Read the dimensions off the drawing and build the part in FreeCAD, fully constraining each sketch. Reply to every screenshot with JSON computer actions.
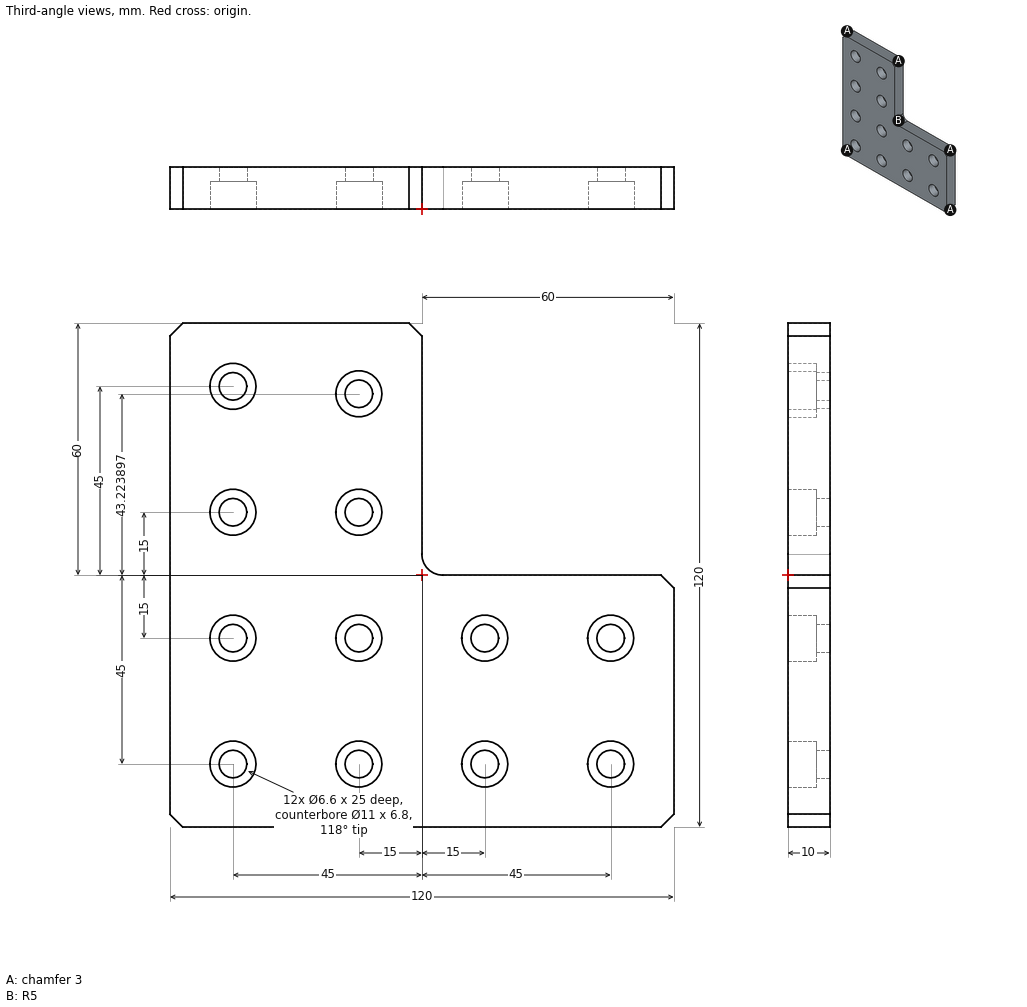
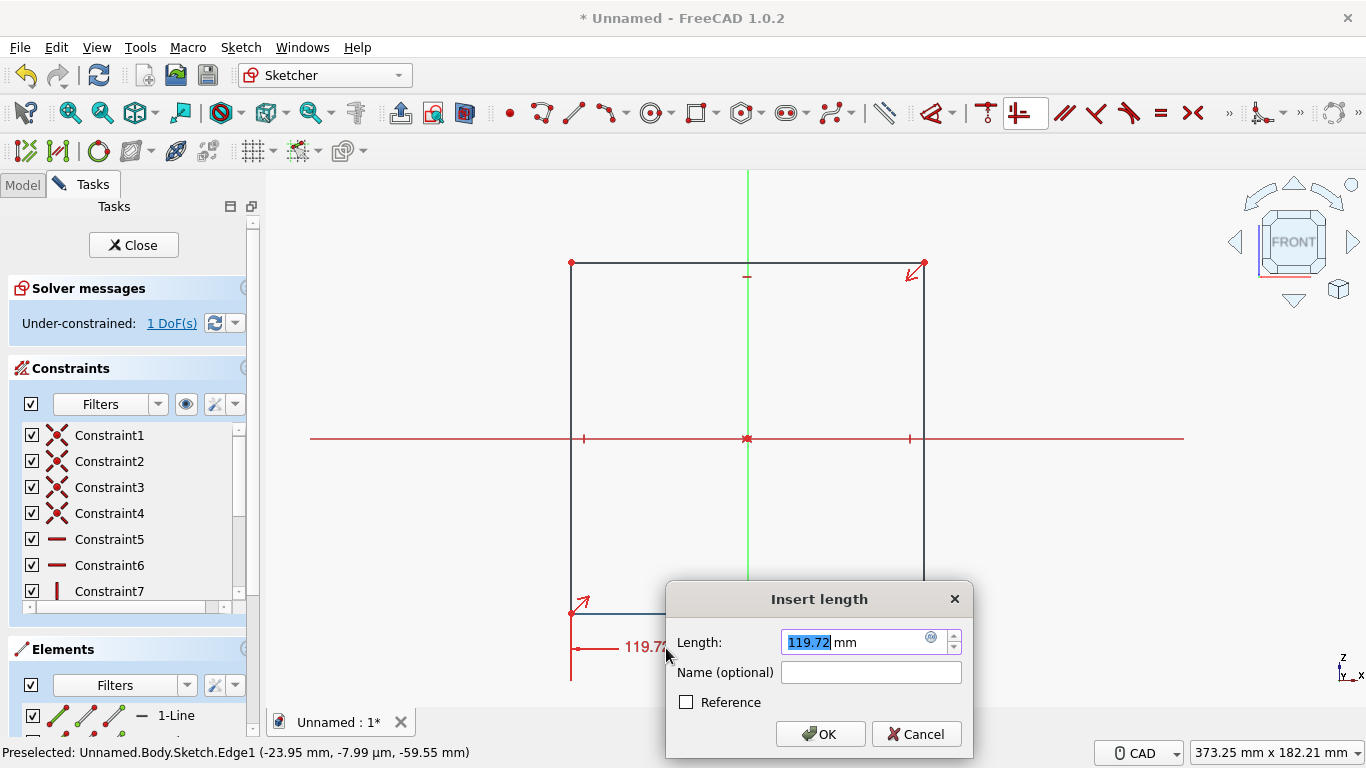
{"action": "type", "text": "120"}
{"action": "key", "text": "Return"}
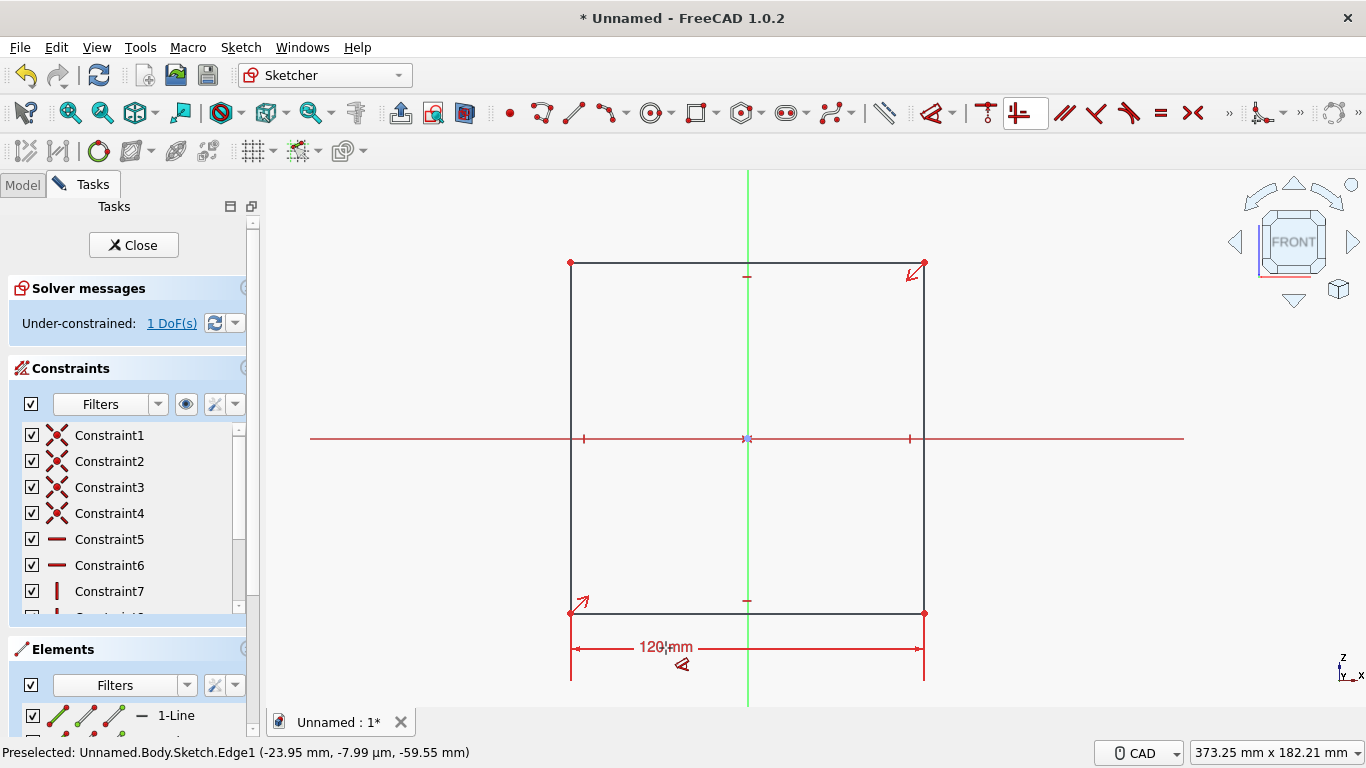
{"action": "left_click", "coordinate": [924, 509]}
{"action": "left_click", "coordinate": [958, 358]}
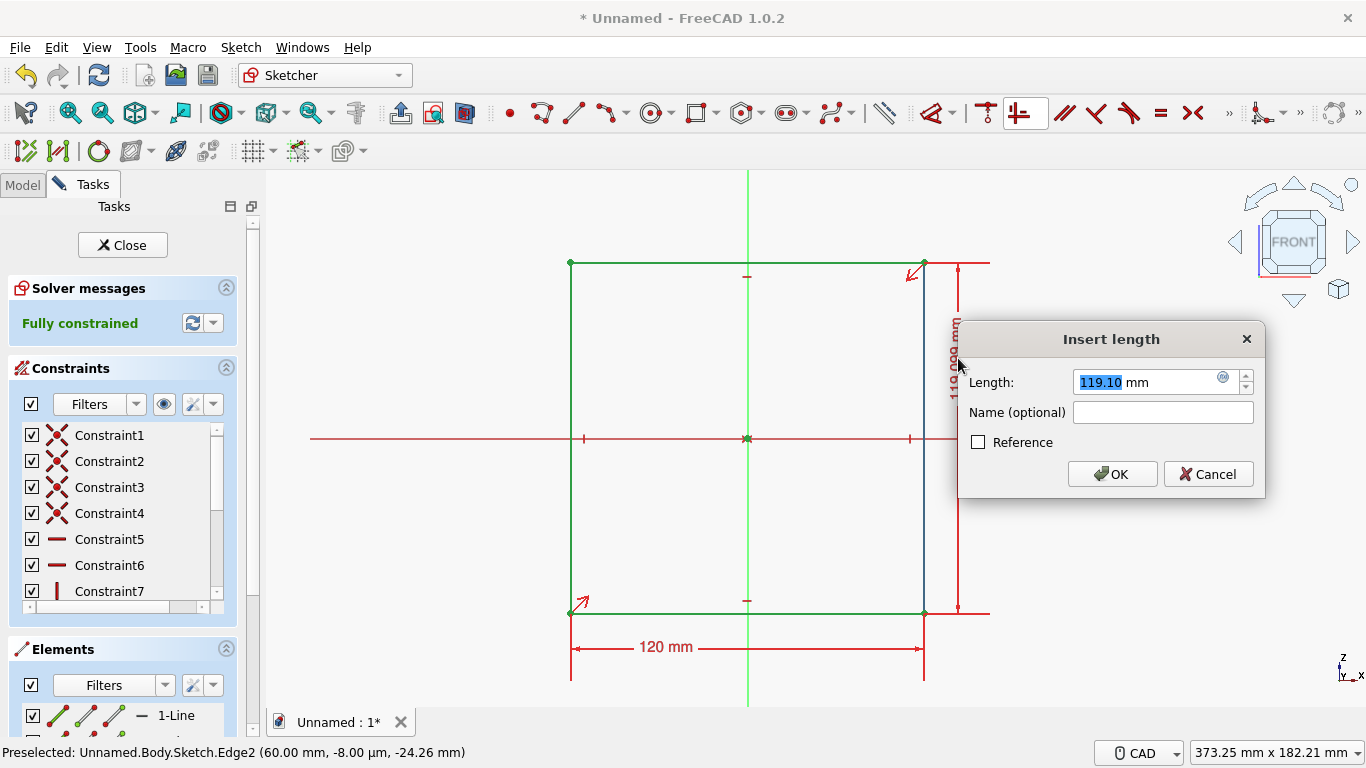
{"action": "type", "text": "120"}
{"action": "key", "text": "Return"}
{"action": "key", "text": "Escape"}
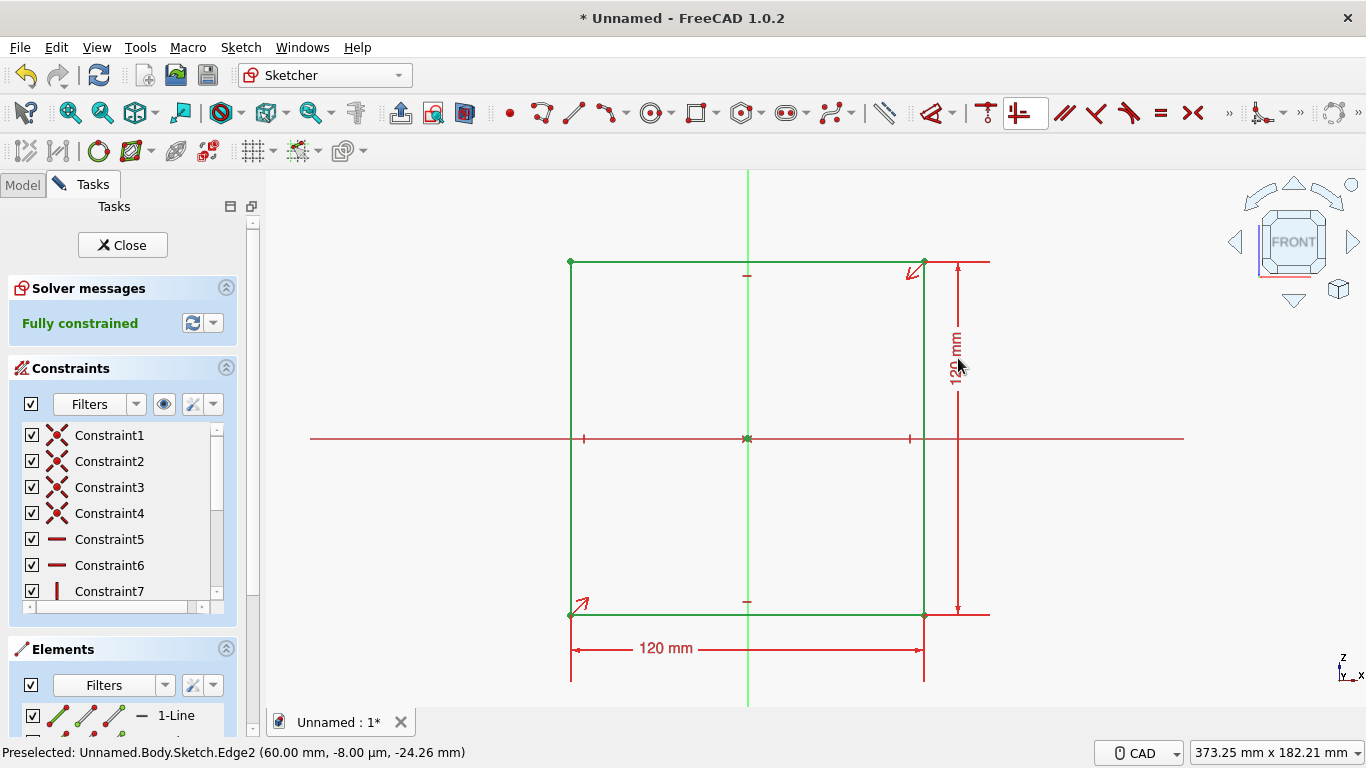
{"action": "left_click", "coordinate": [123, 245]}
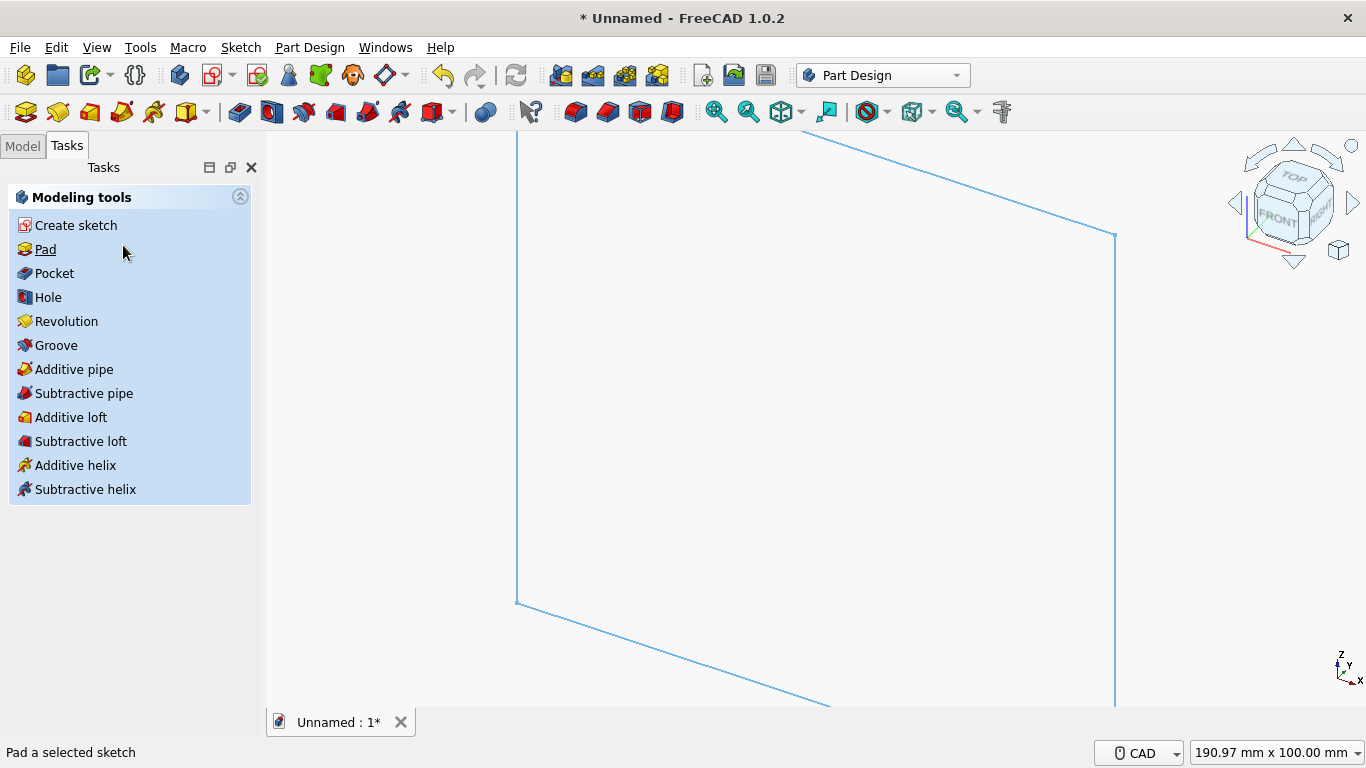
{"action": "left_click", "coordinate": [26, 112]}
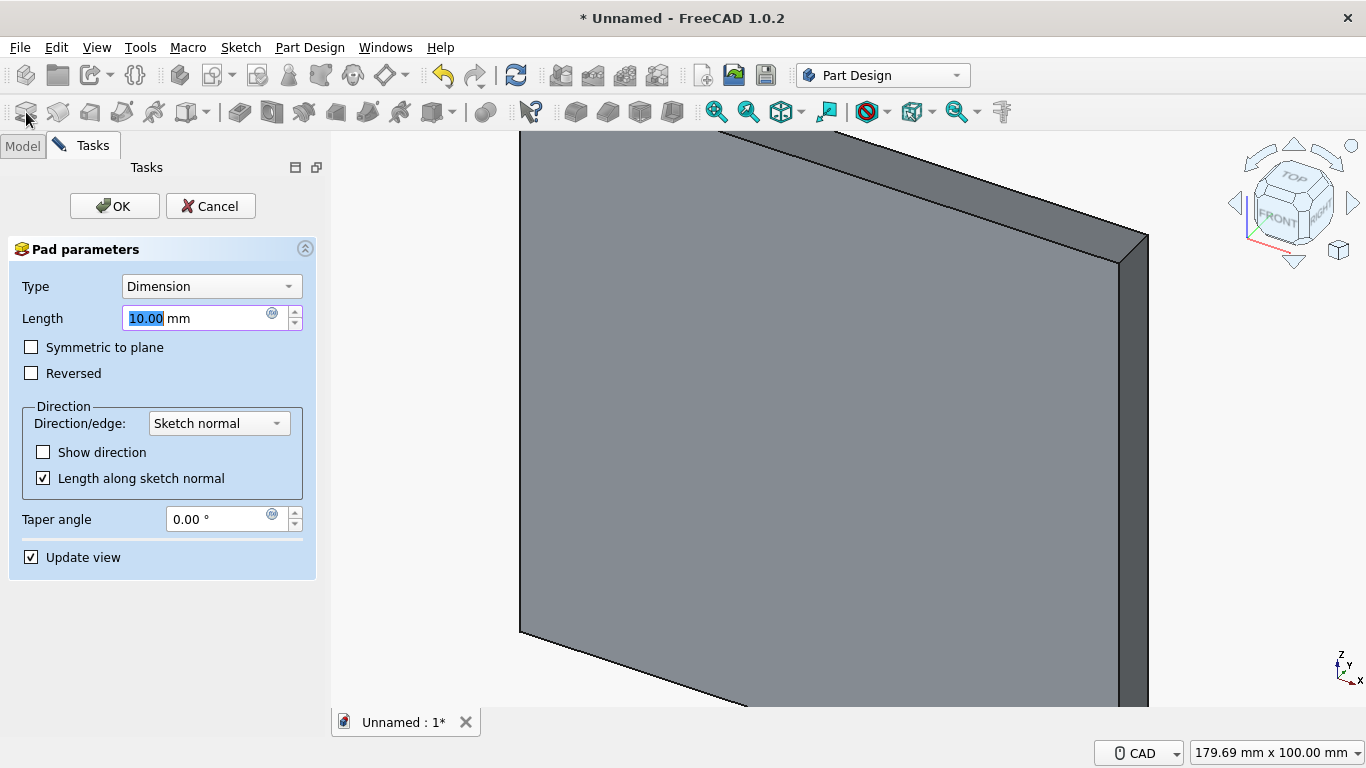
{"action": "type", "text": "10"}
{"action": "key", "text": "Tab"}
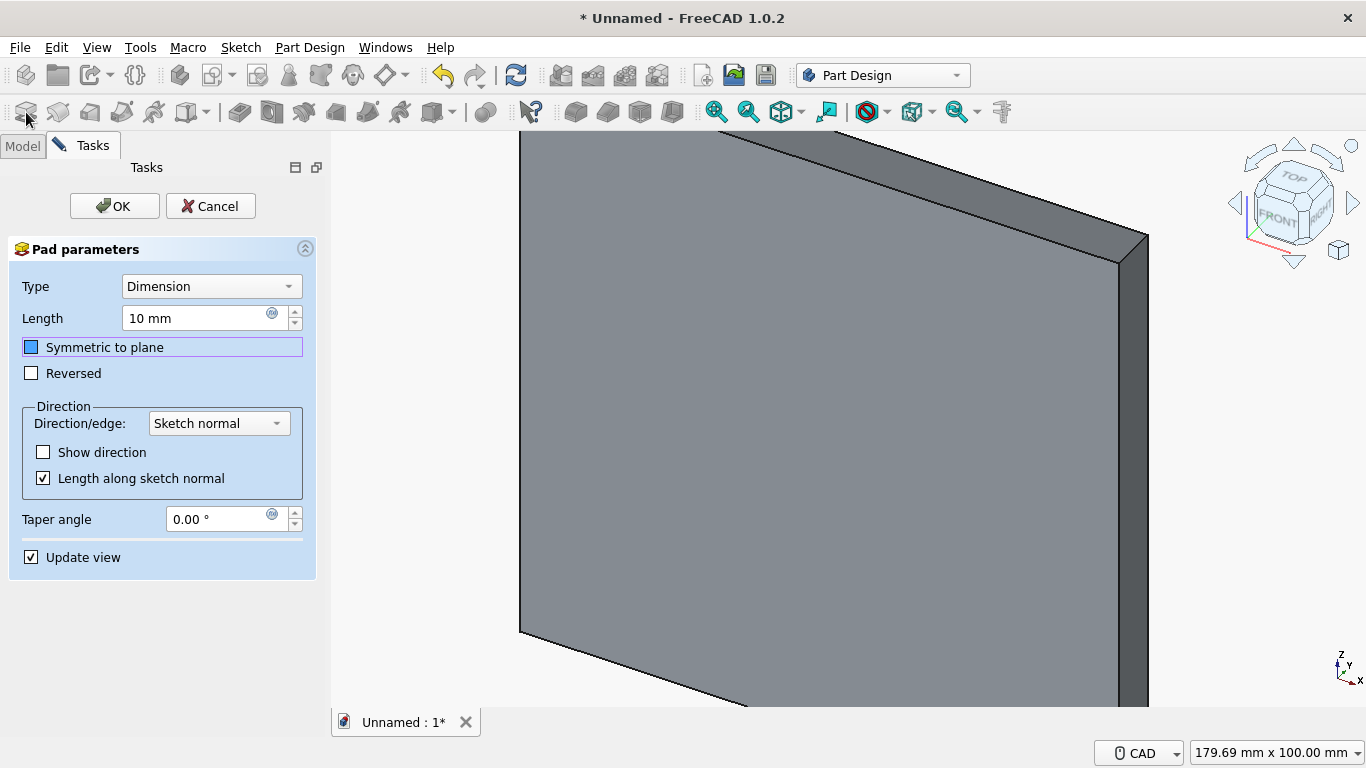
{"action": "left_click", "coordinate": [30, 373]}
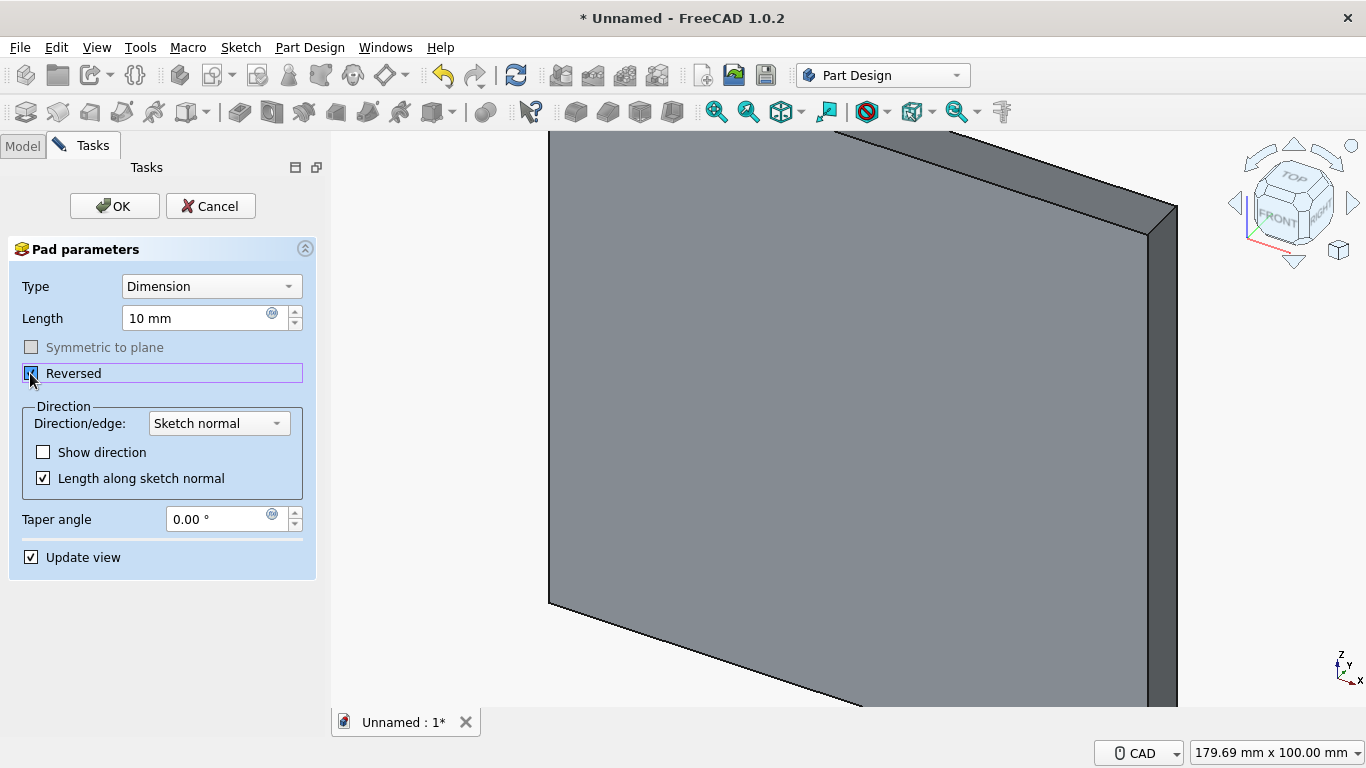
{"action": "left_click", "coordinate": [115, 206]}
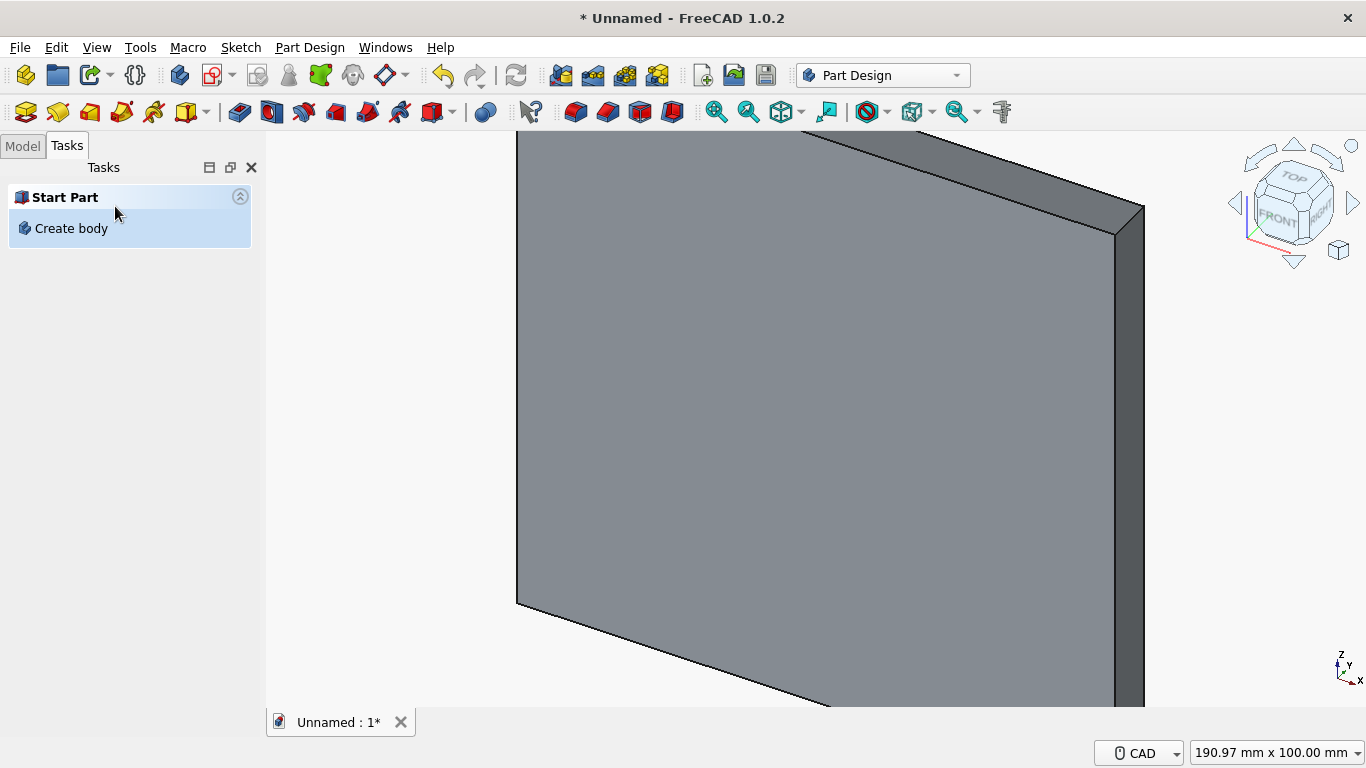
{"action": "left_click", "coordinate": [718, 112]}